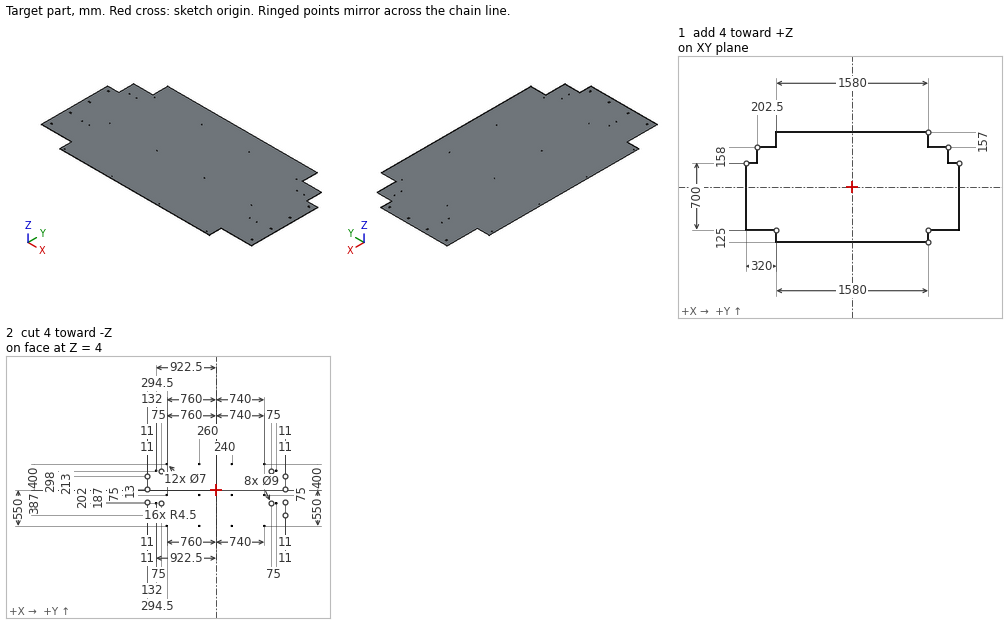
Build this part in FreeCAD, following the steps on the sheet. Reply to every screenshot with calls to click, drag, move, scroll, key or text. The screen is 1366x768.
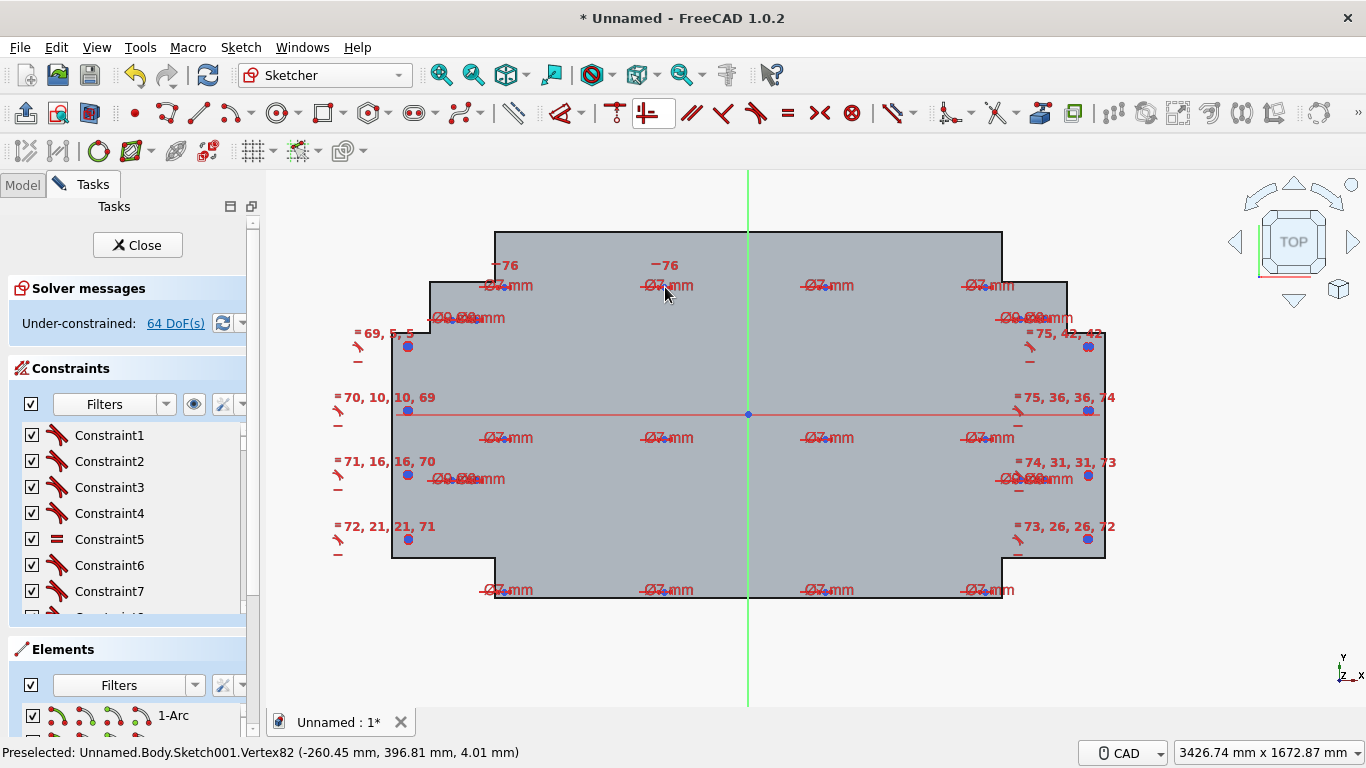
click(665, 287)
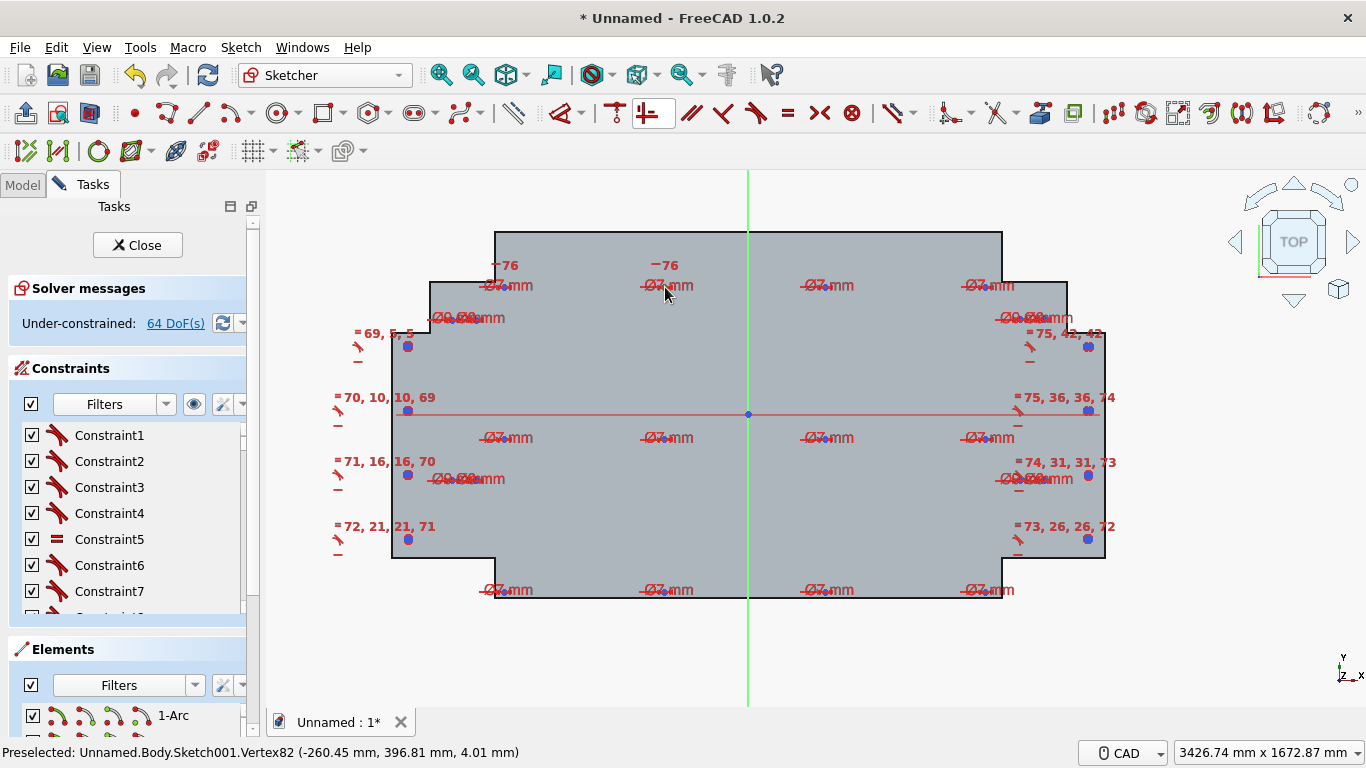
click(825, 287)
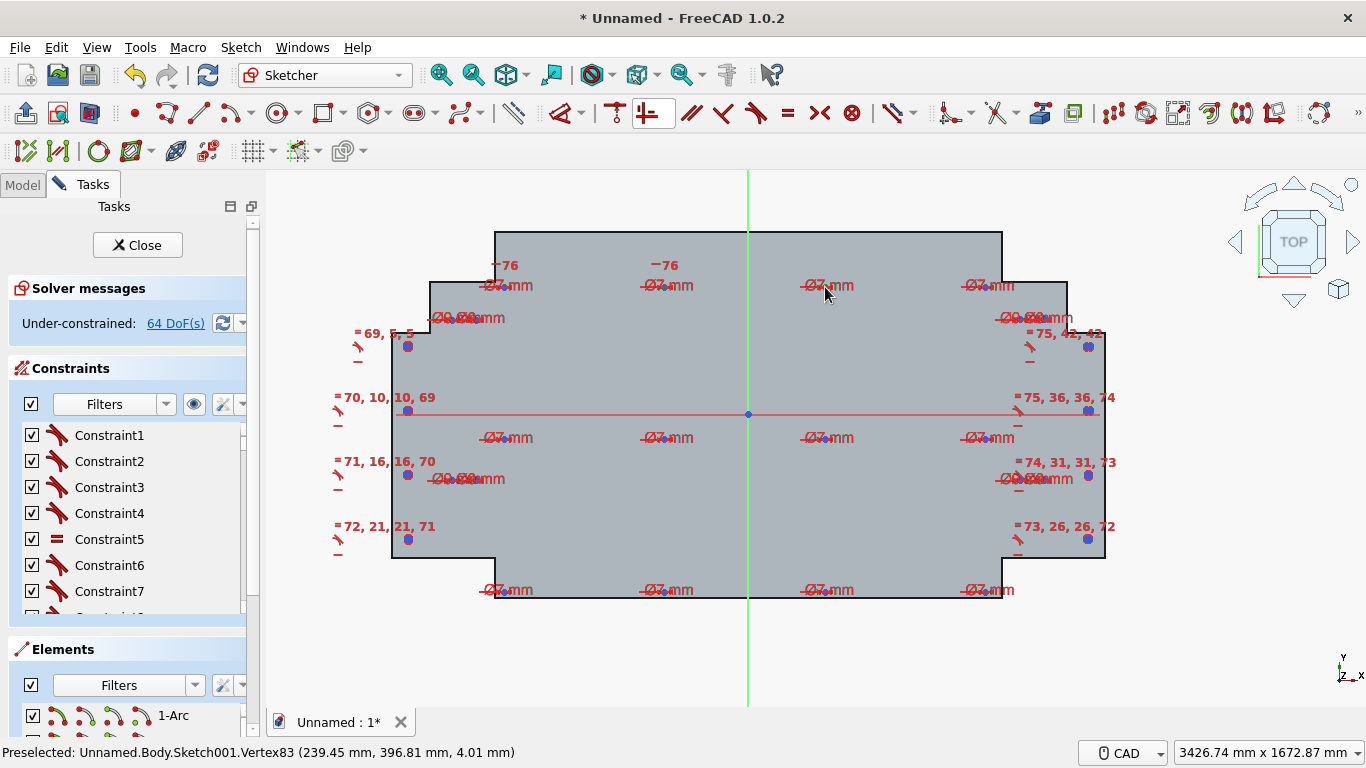
click(670, 114)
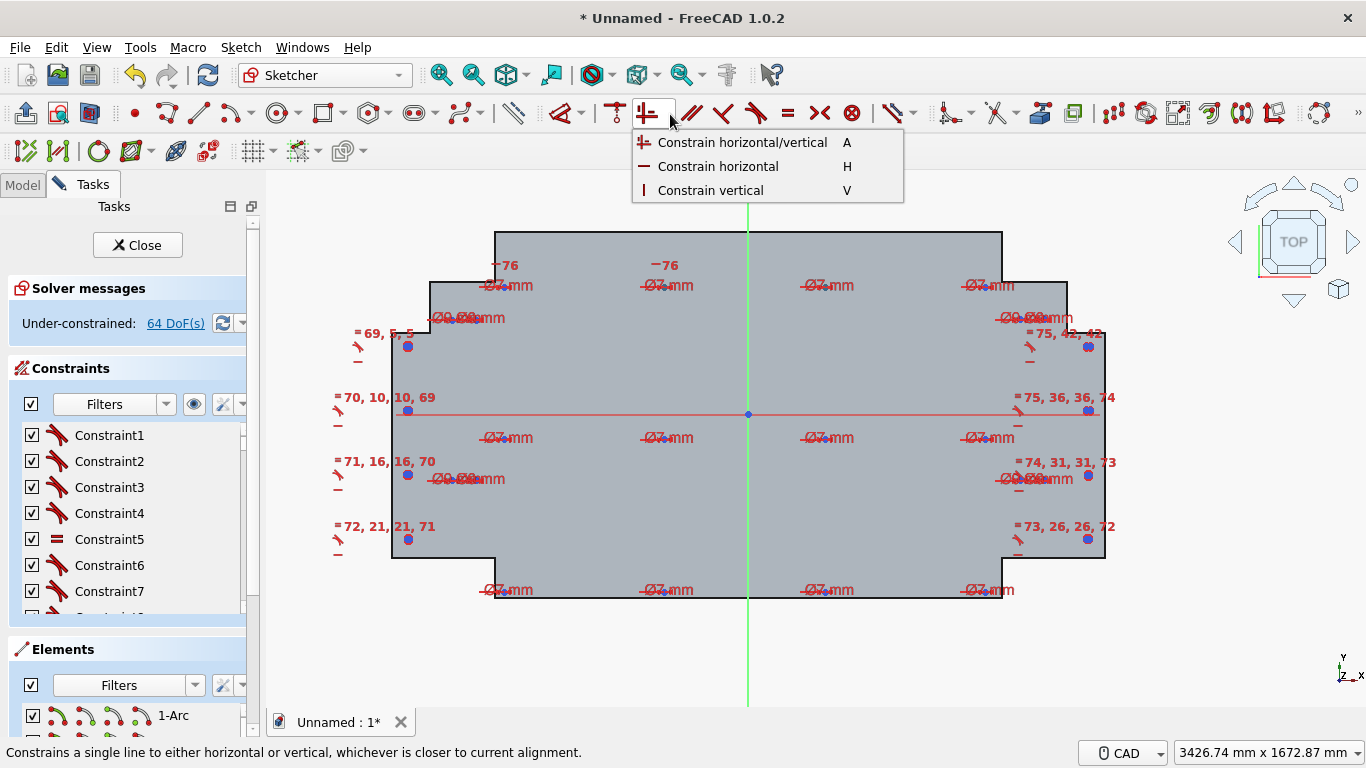
click(768, 166)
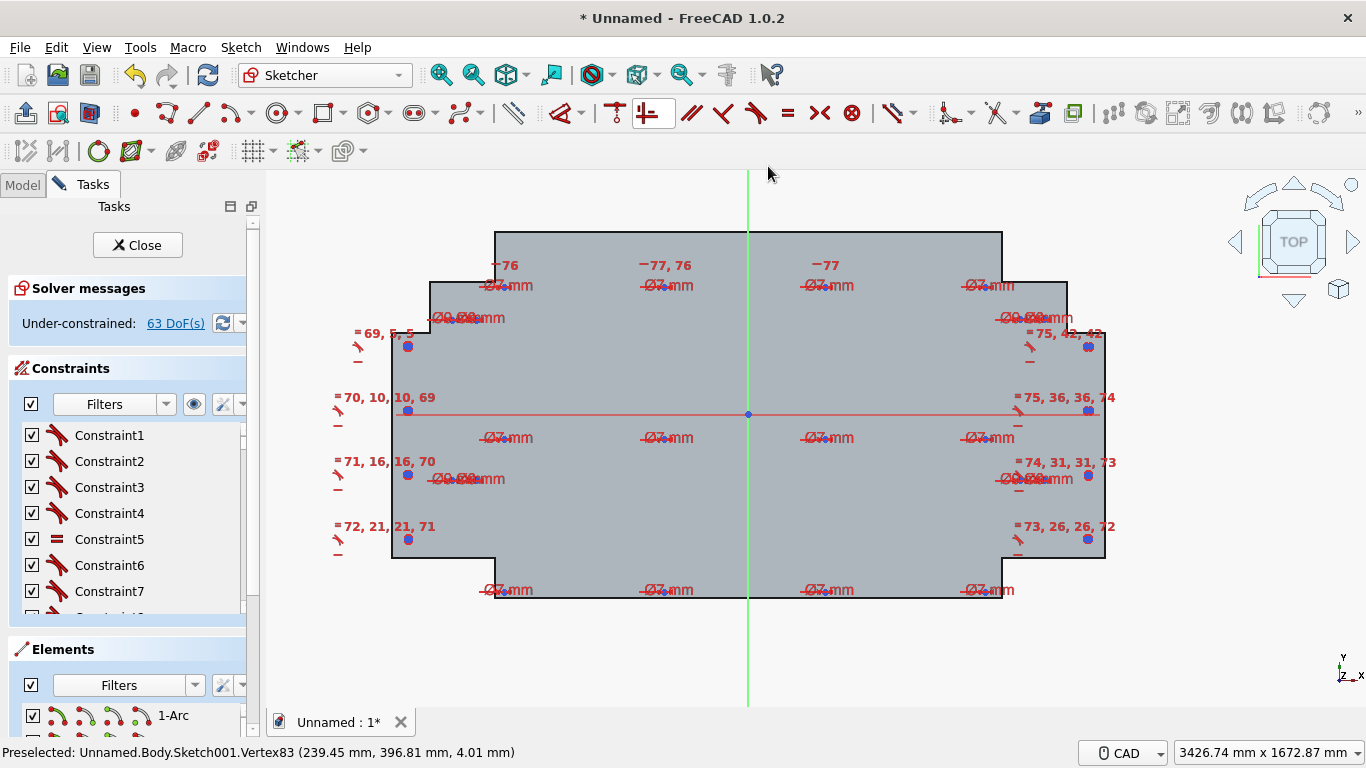
click(665, 287)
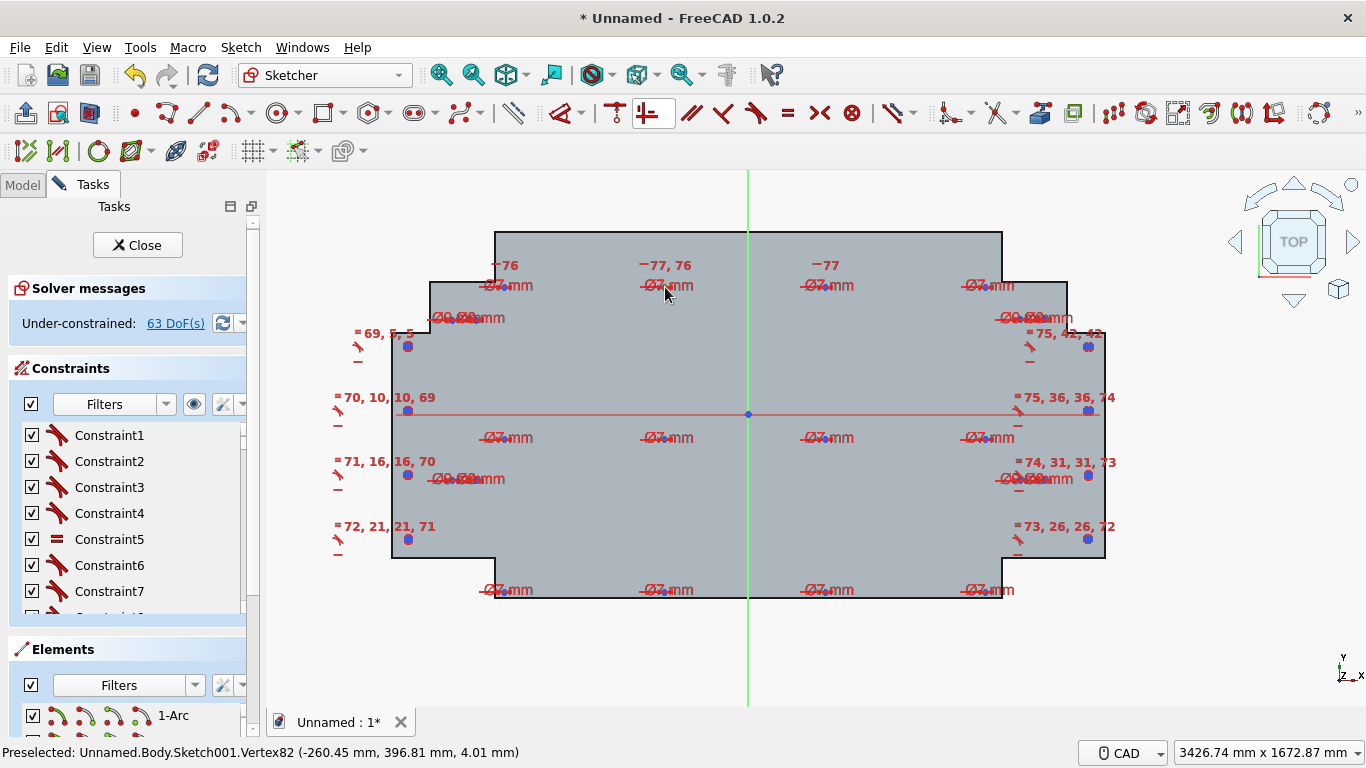
click(665, 440)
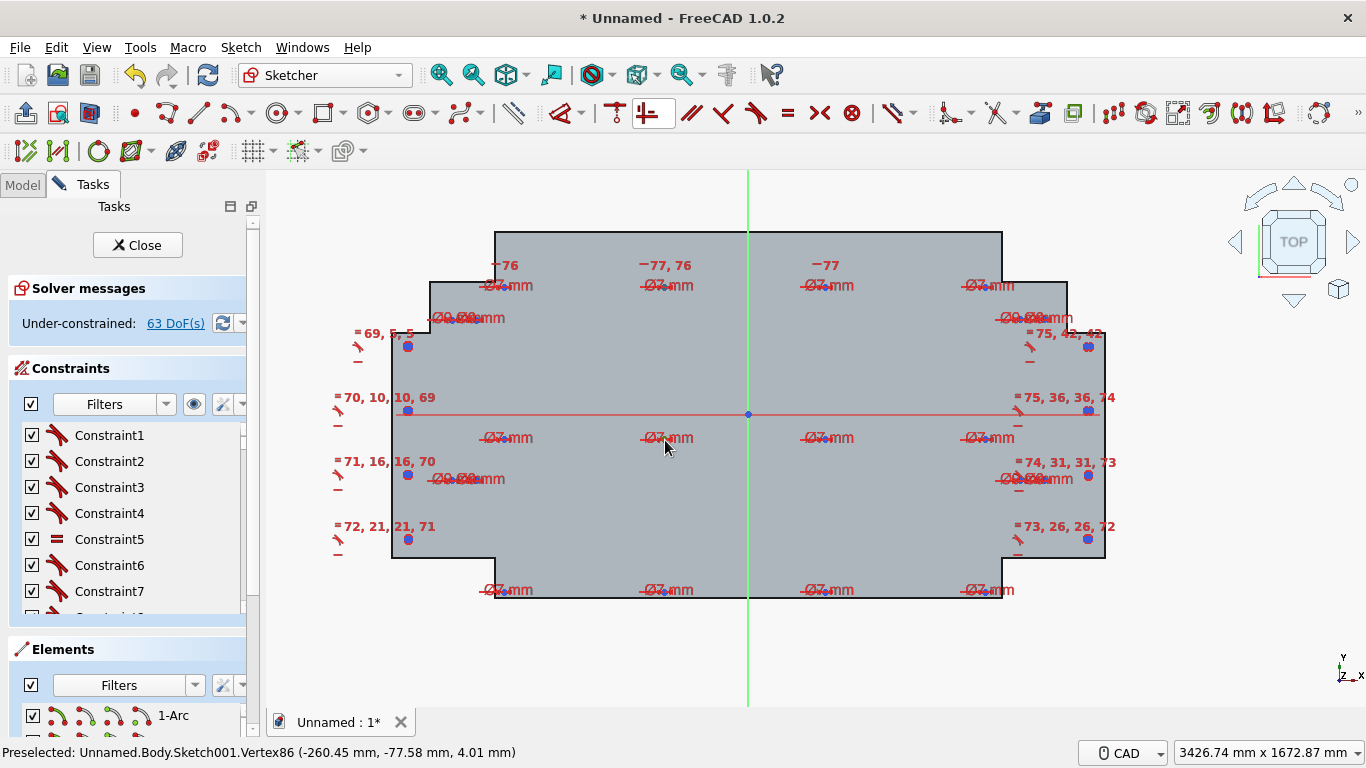
key(v)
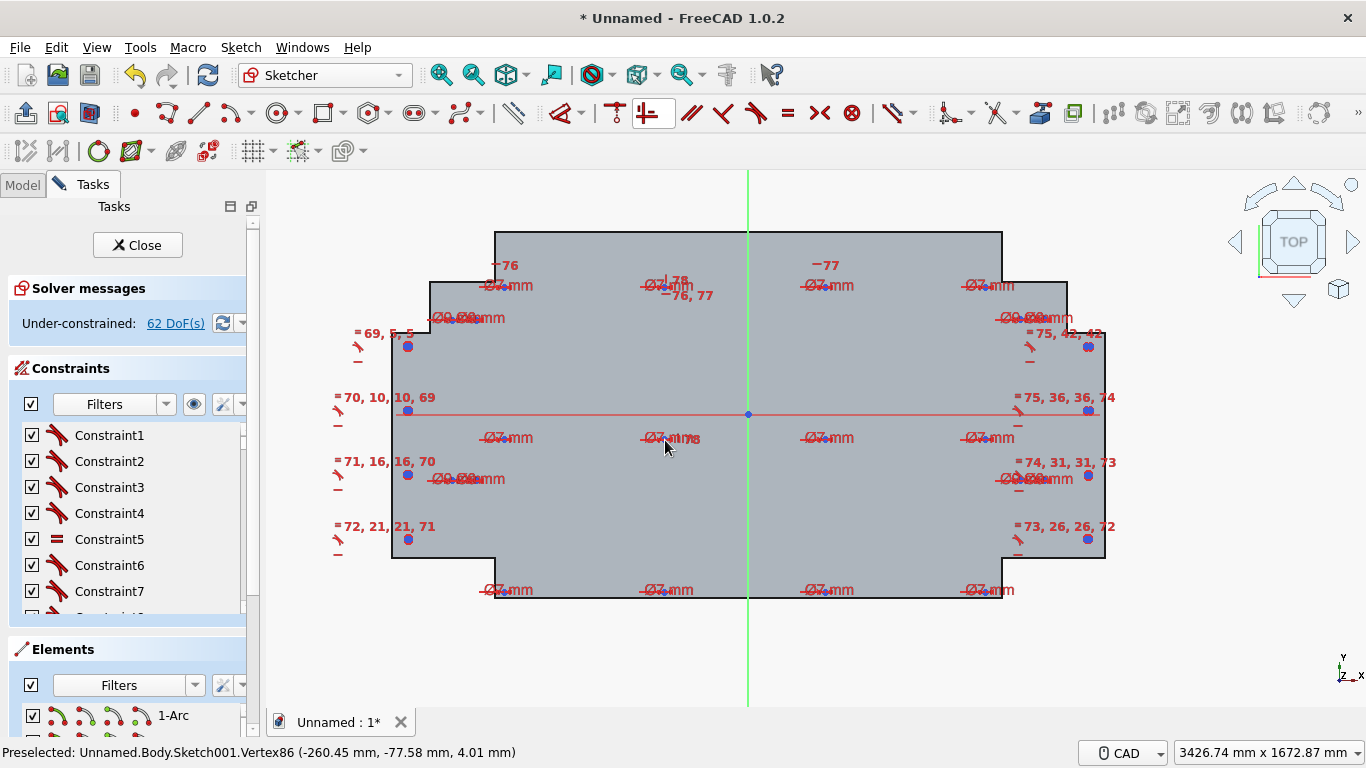
click(504, 440)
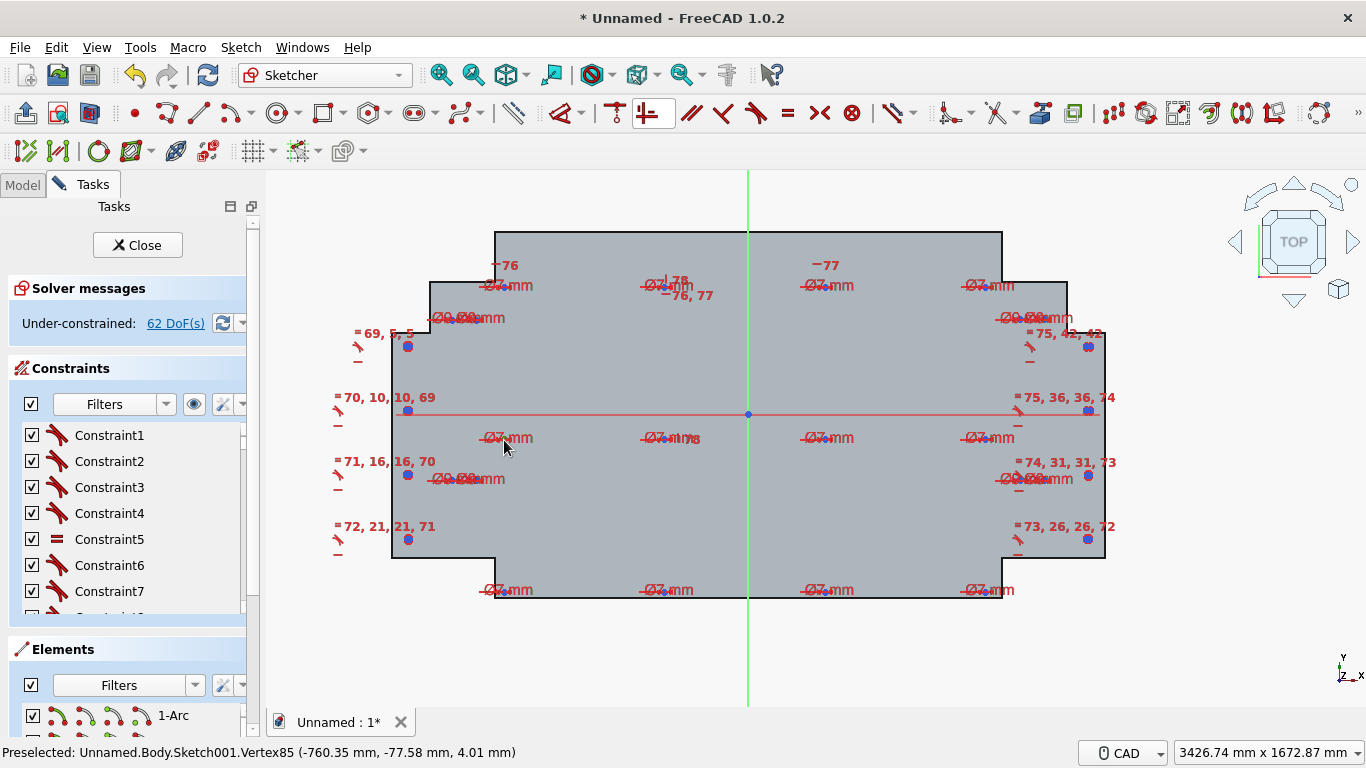
click(665, 440)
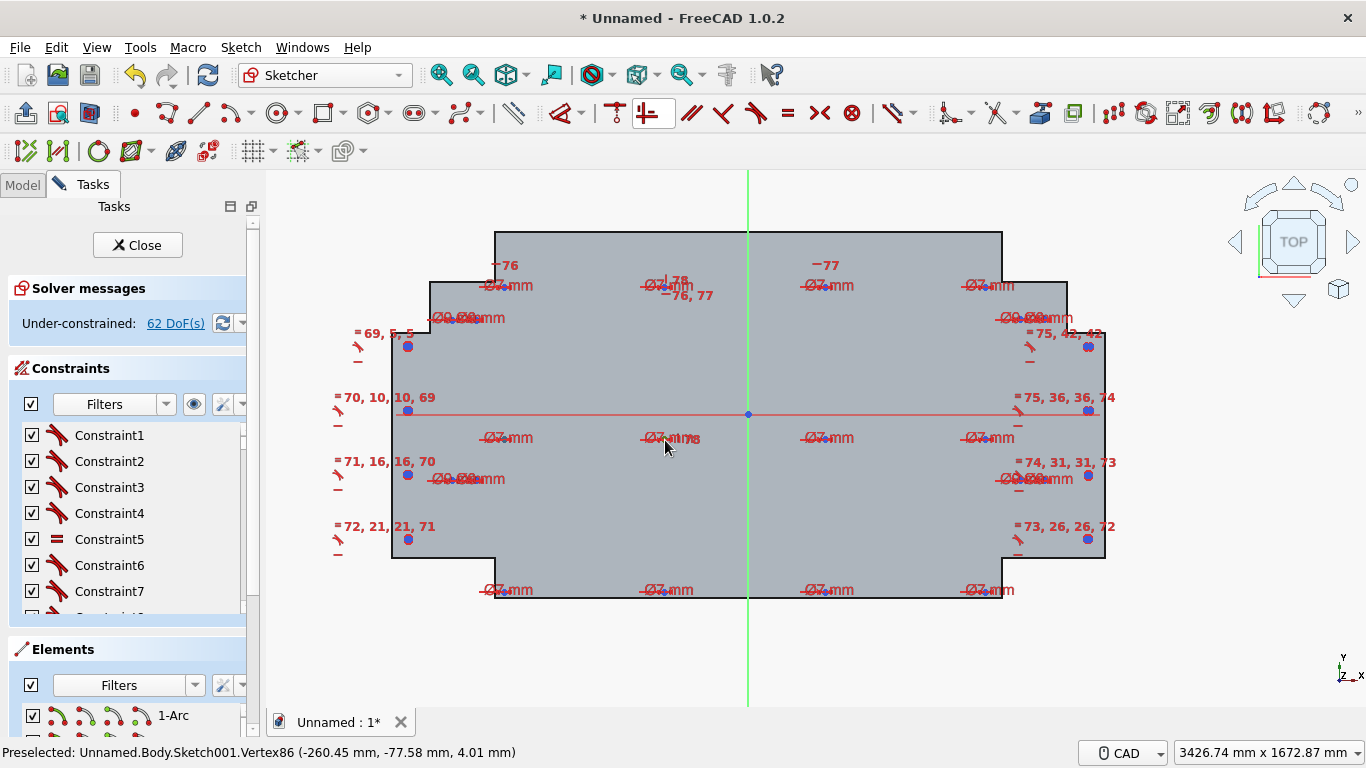
click(670, 114)